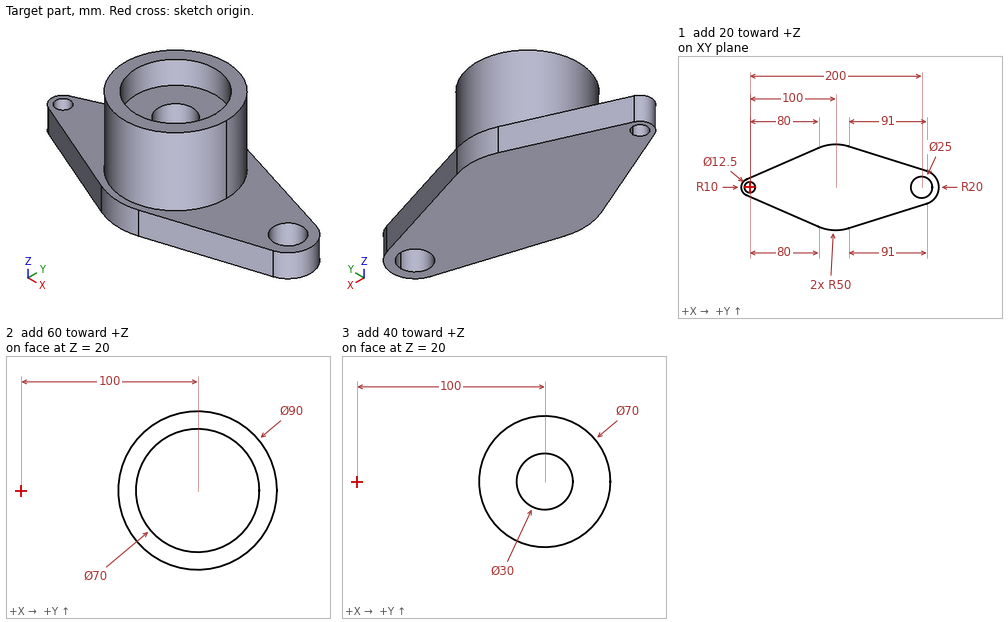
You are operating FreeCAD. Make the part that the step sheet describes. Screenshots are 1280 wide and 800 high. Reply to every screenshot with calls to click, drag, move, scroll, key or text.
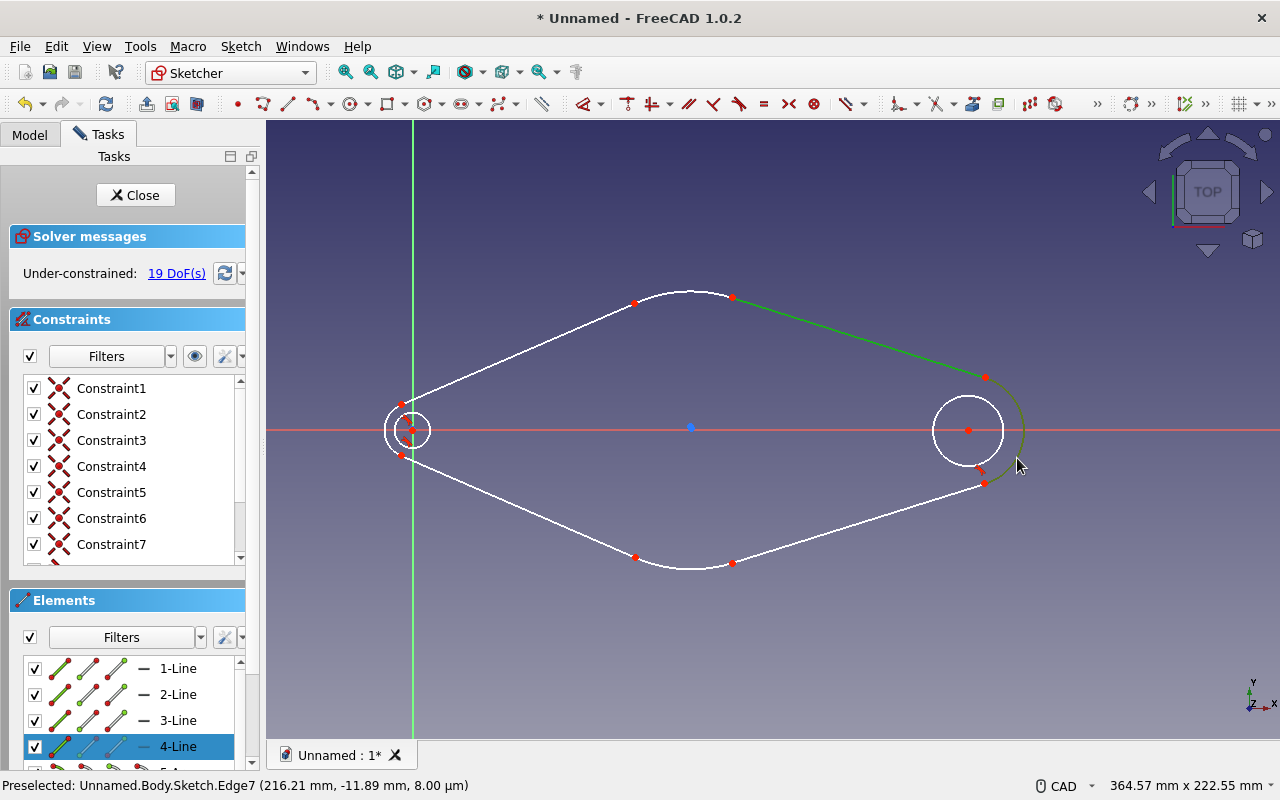
click(739, 104)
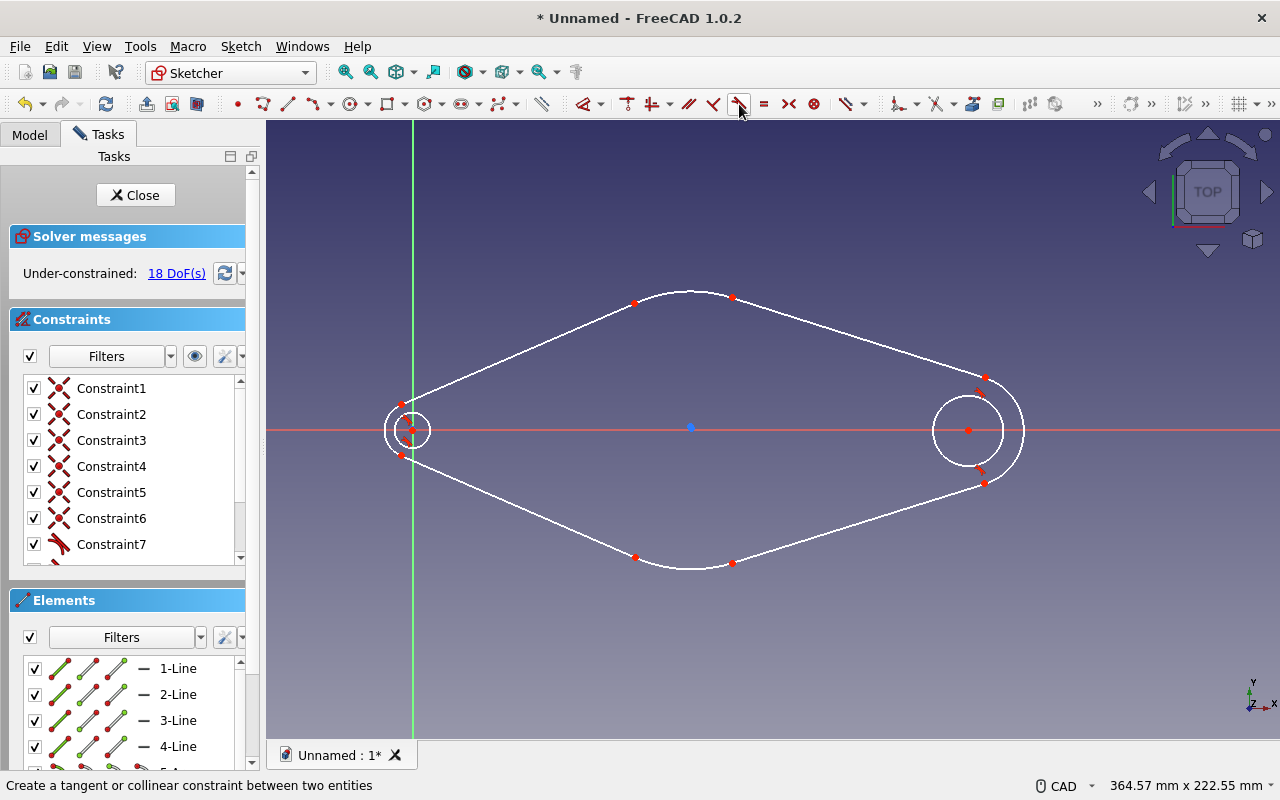
click(664, 567)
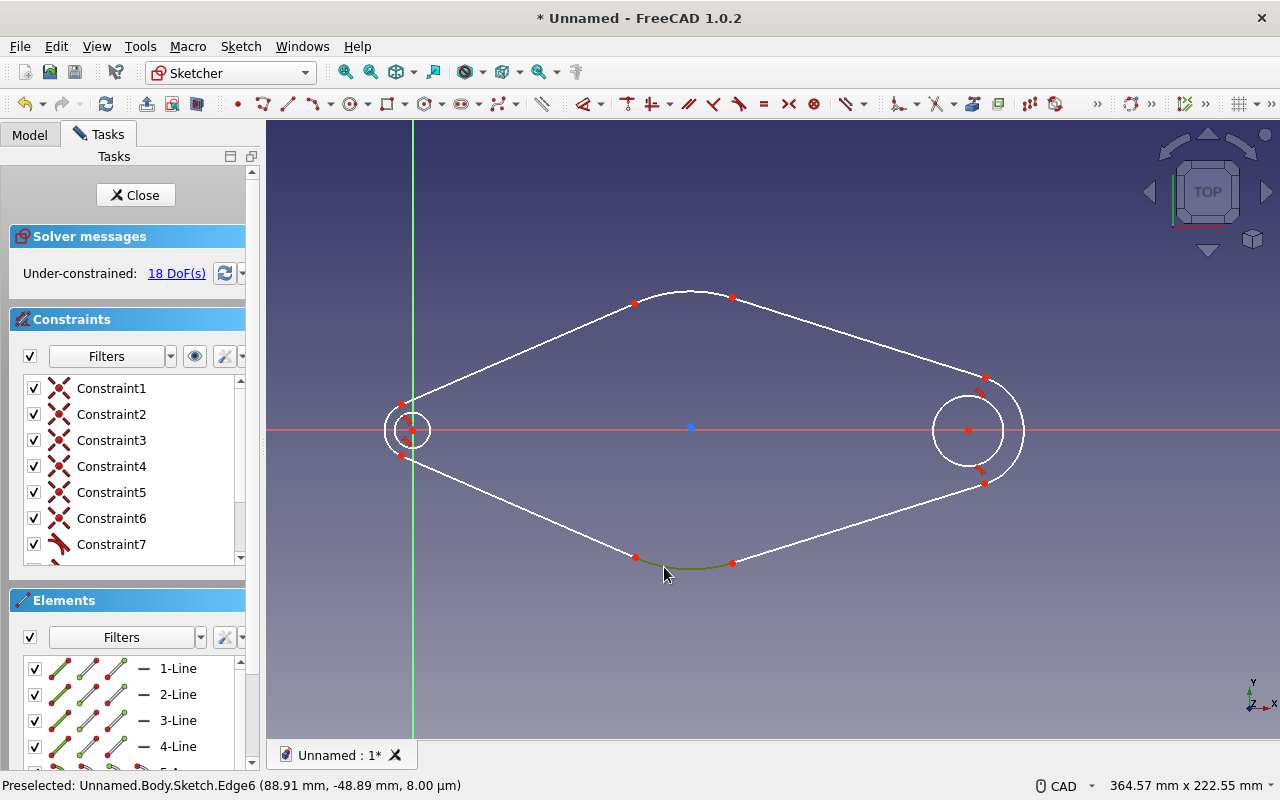
click(703, 292)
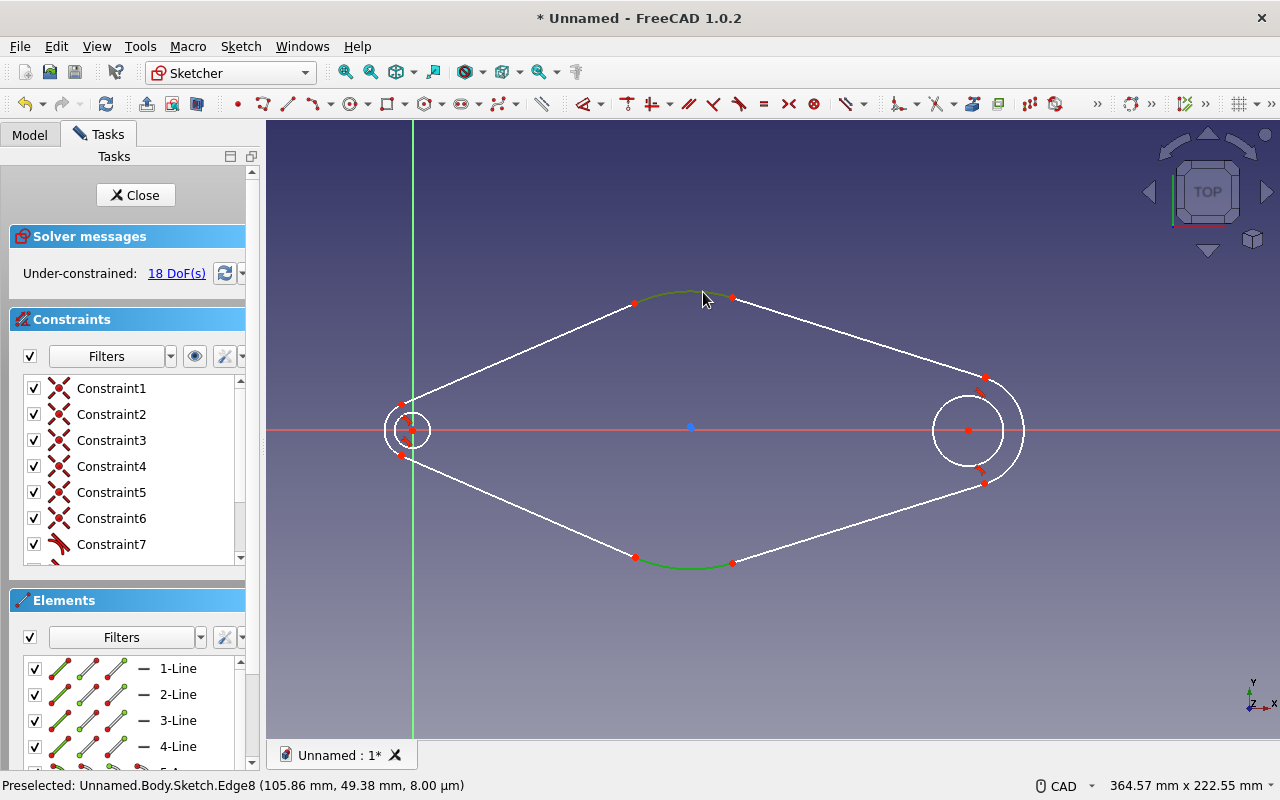
click(627, 104)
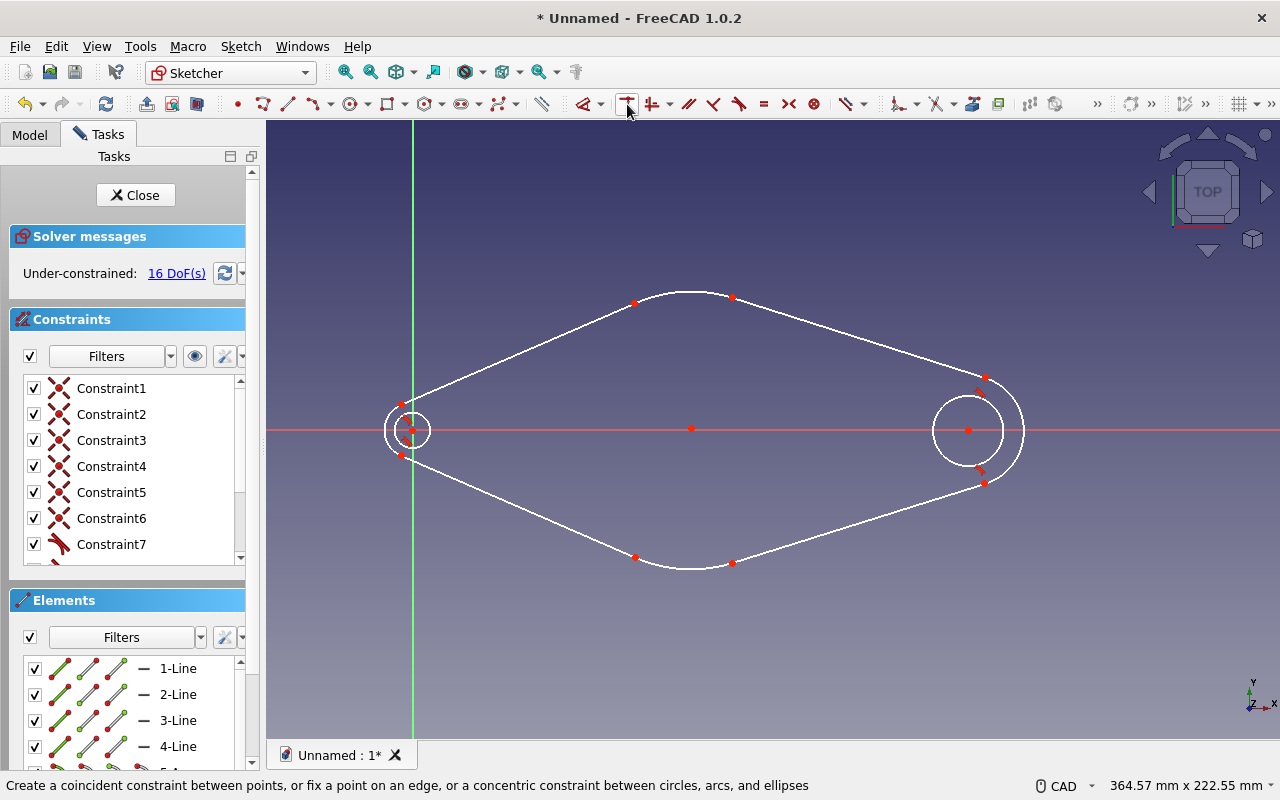
scroll(412, 430, up, 5)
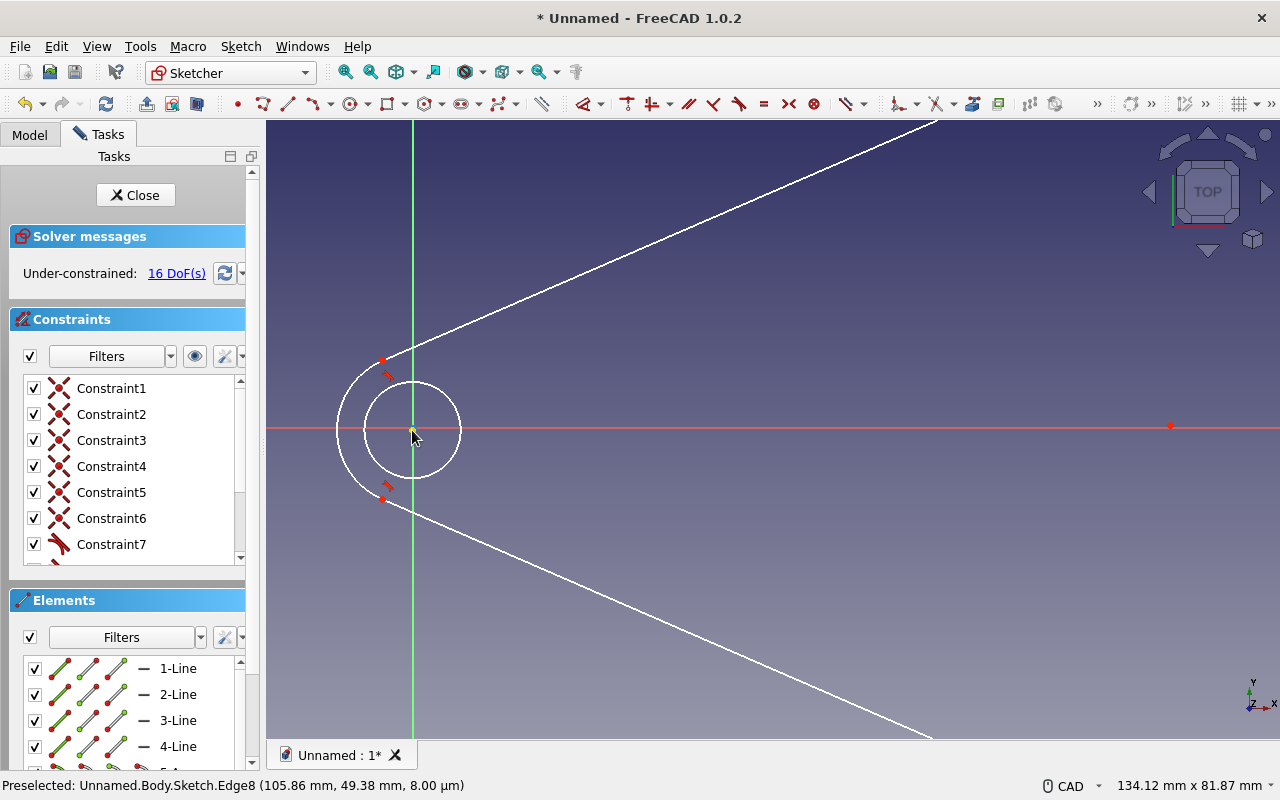
drag(403, 418, 423, 440)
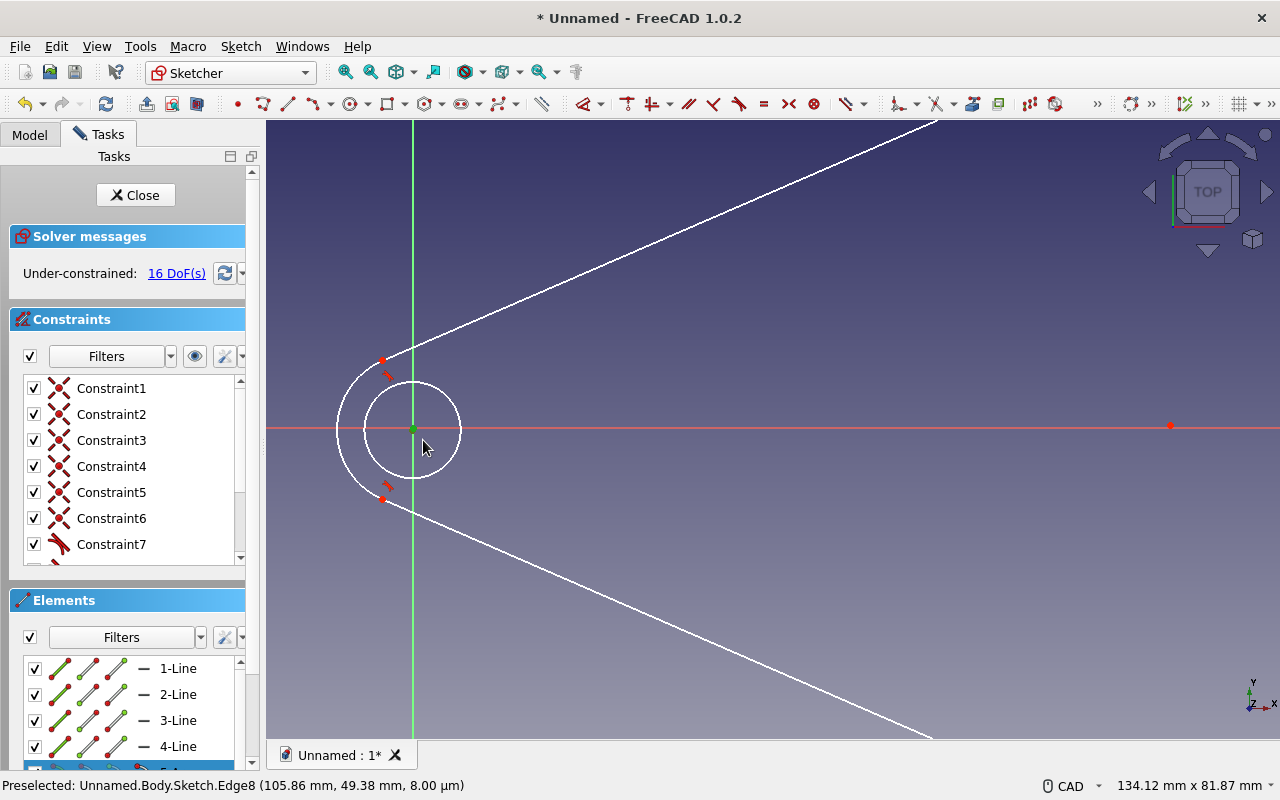
click(627, 104)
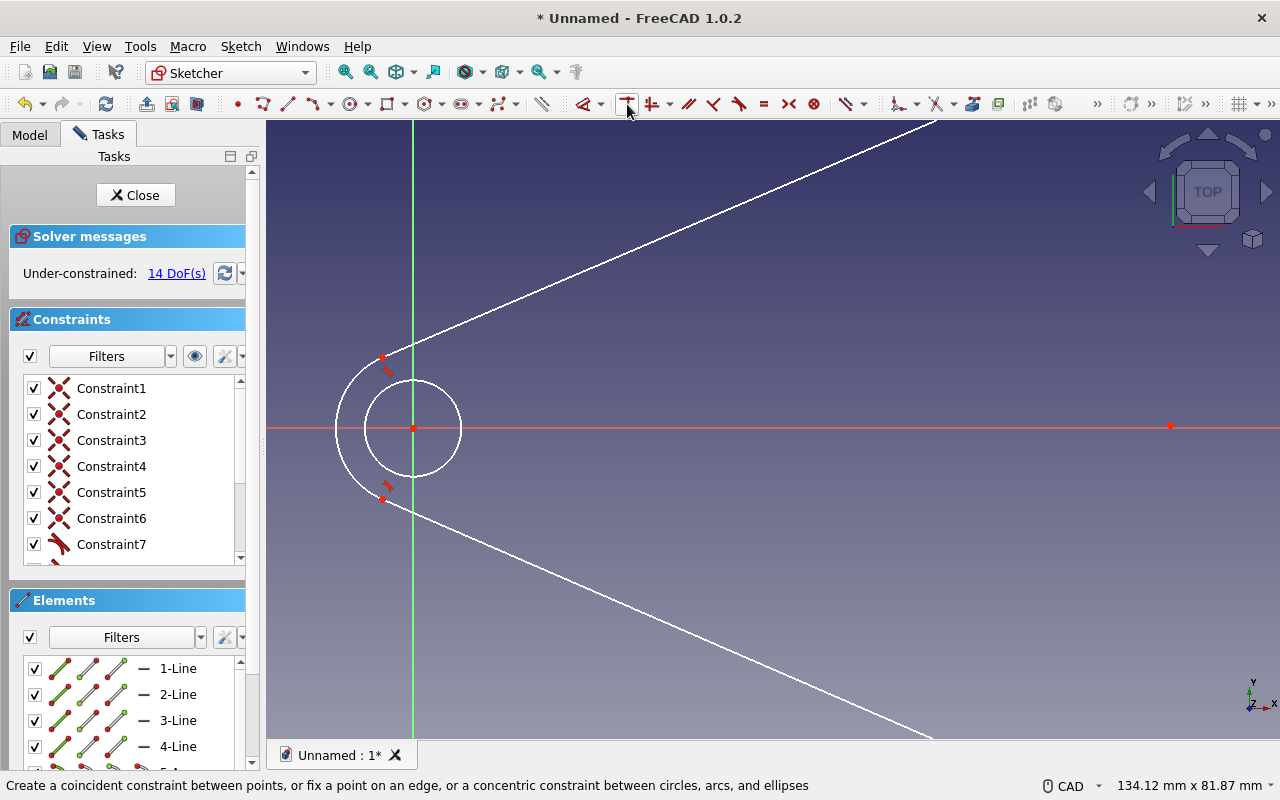
scroll(412, 430, down, 5)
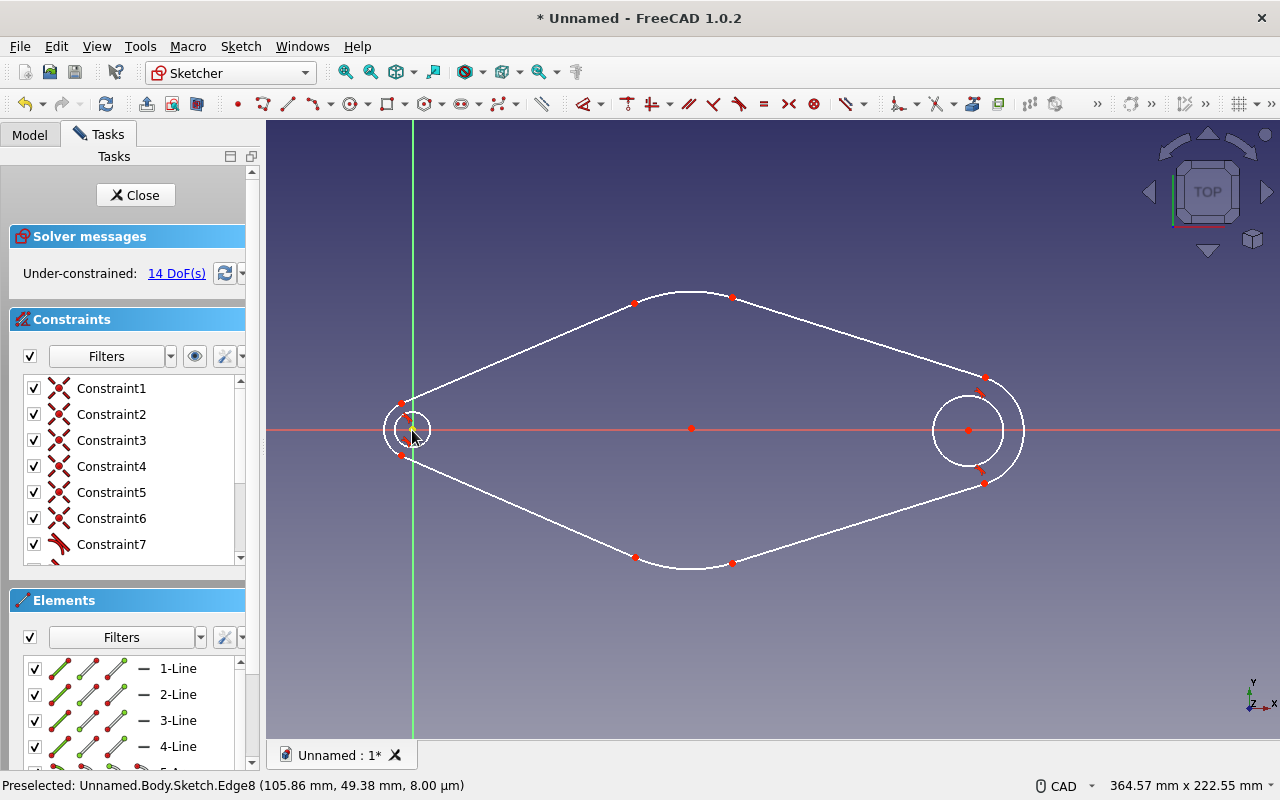
click(664, 567)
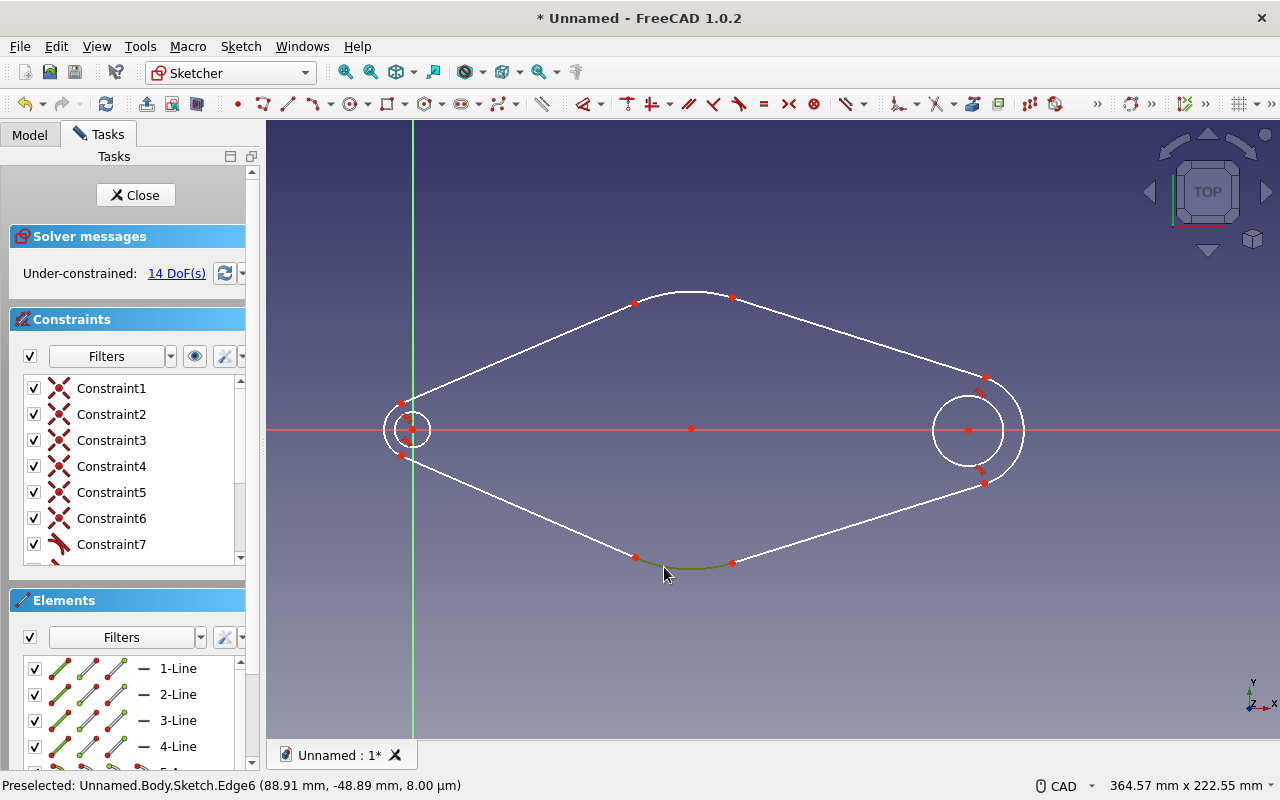
click(703, 292)